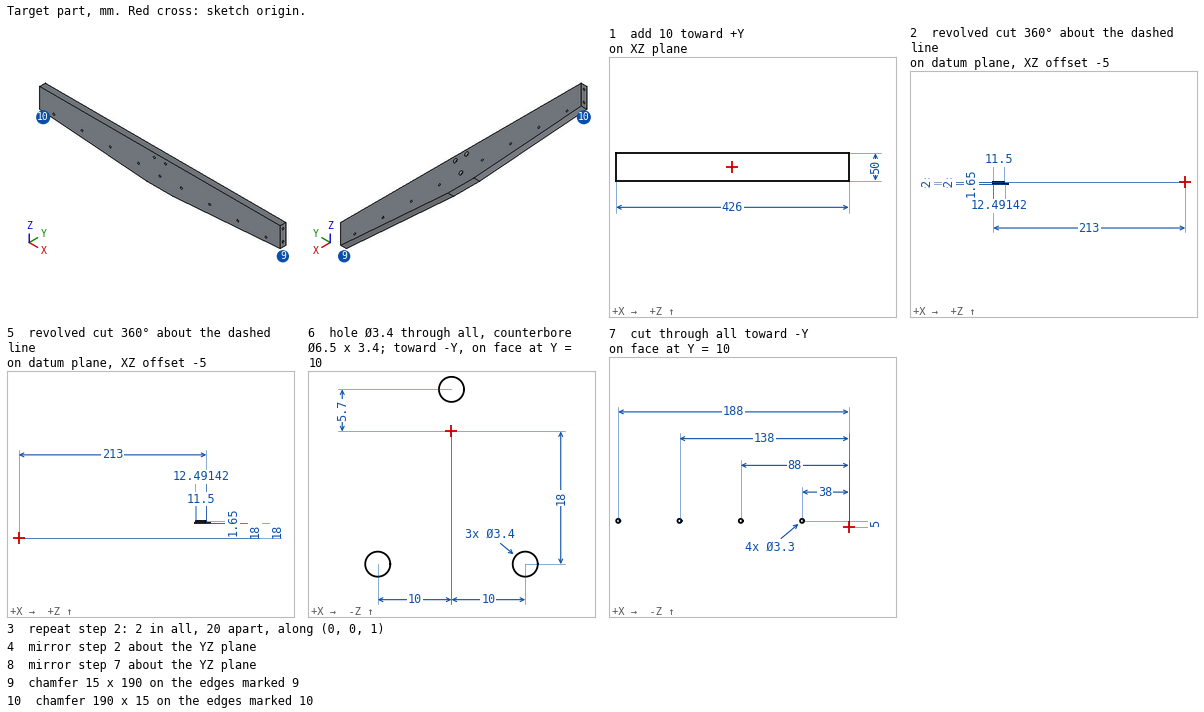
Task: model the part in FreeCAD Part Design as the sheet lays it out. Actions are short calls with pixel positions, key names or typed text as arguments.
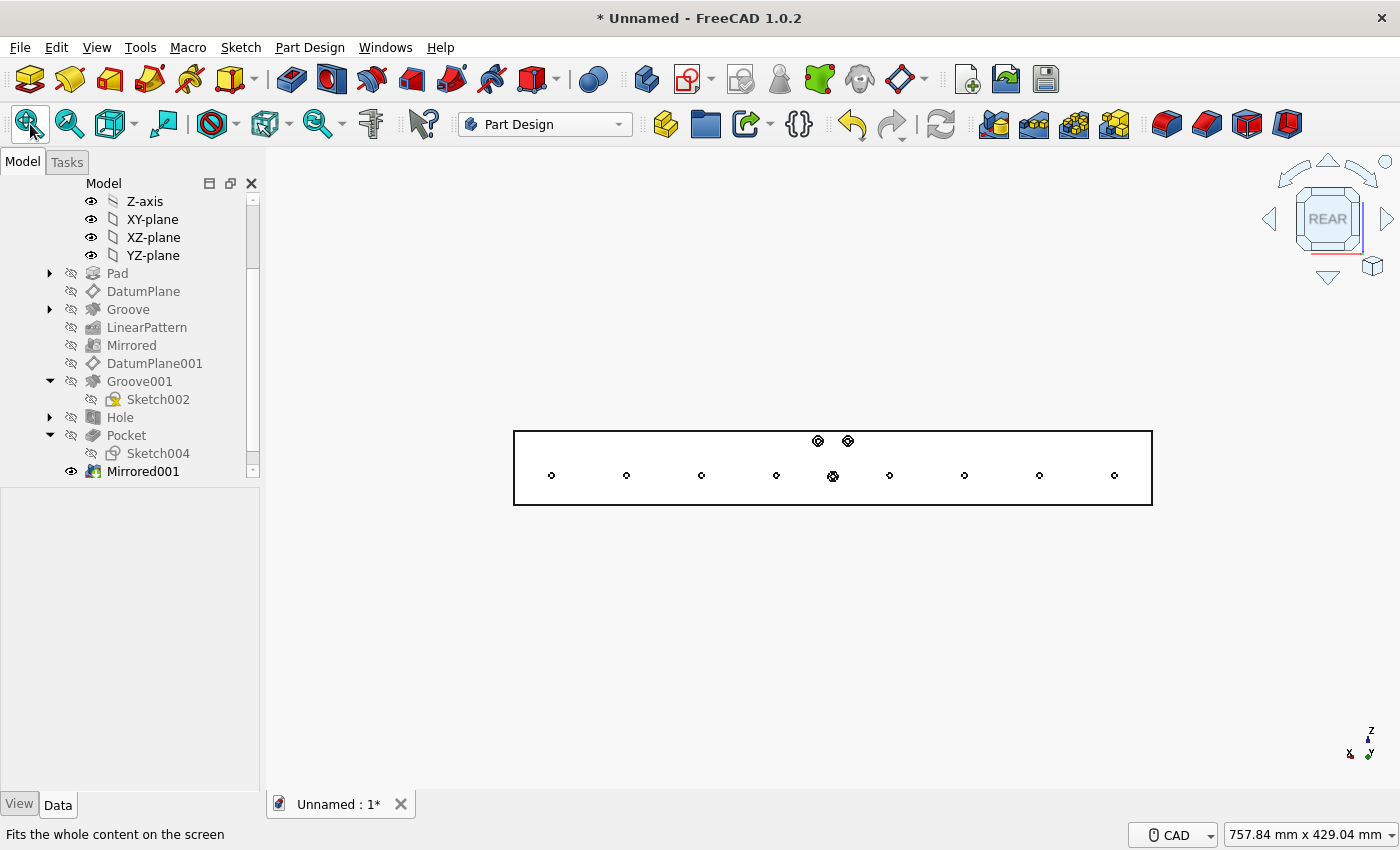
key(0)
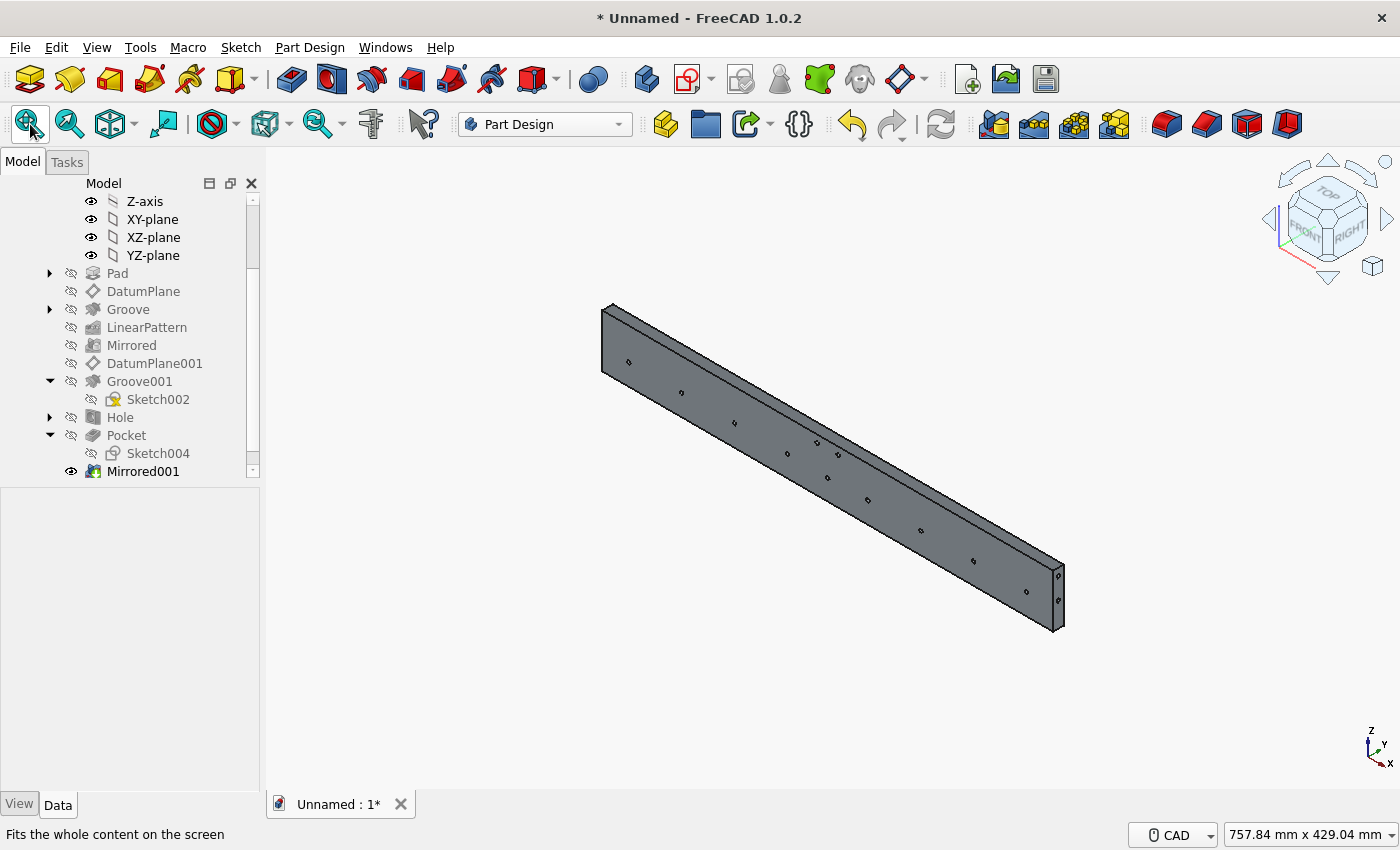
scroll(1058, 628, up, 5)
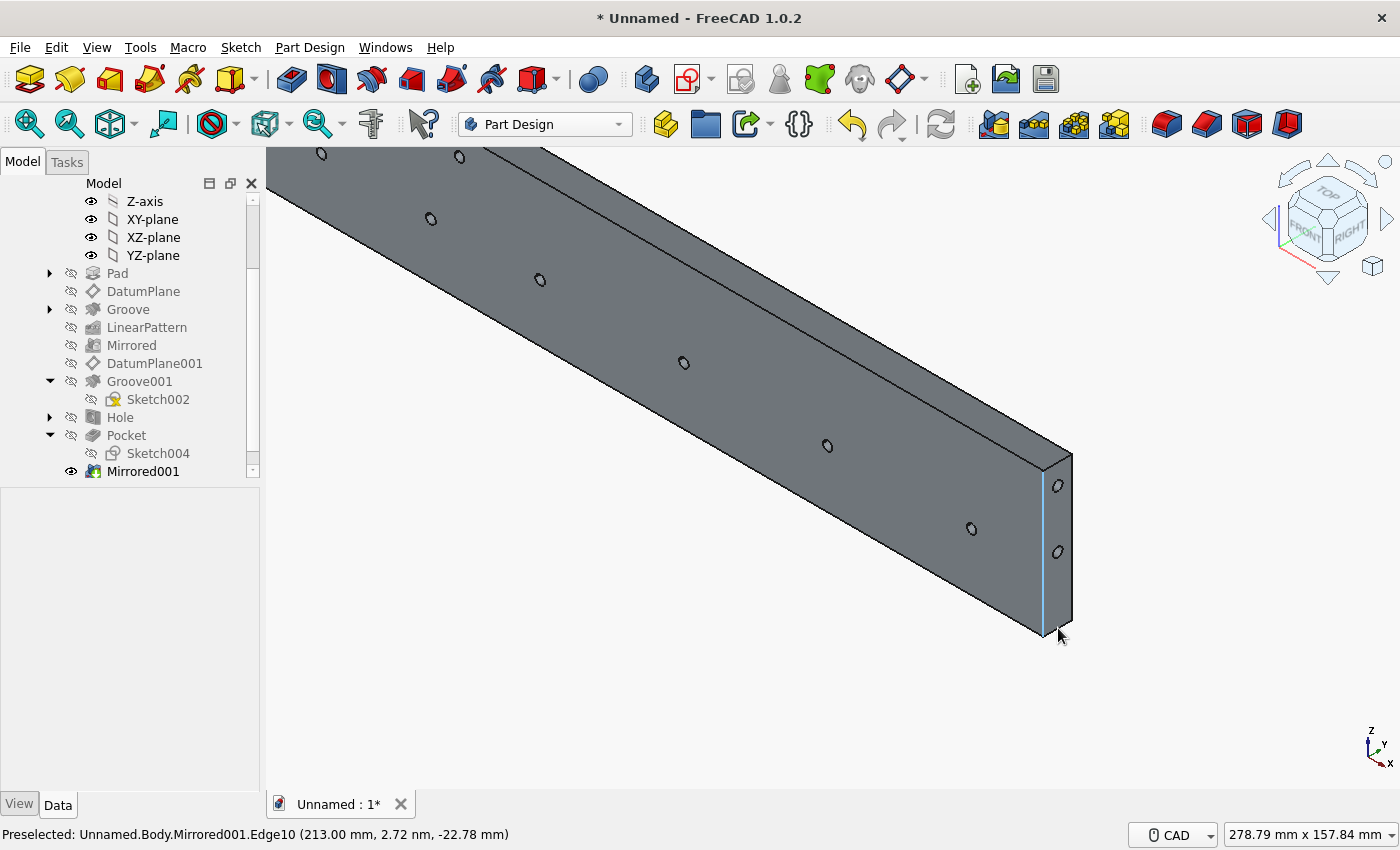
click(30, 124)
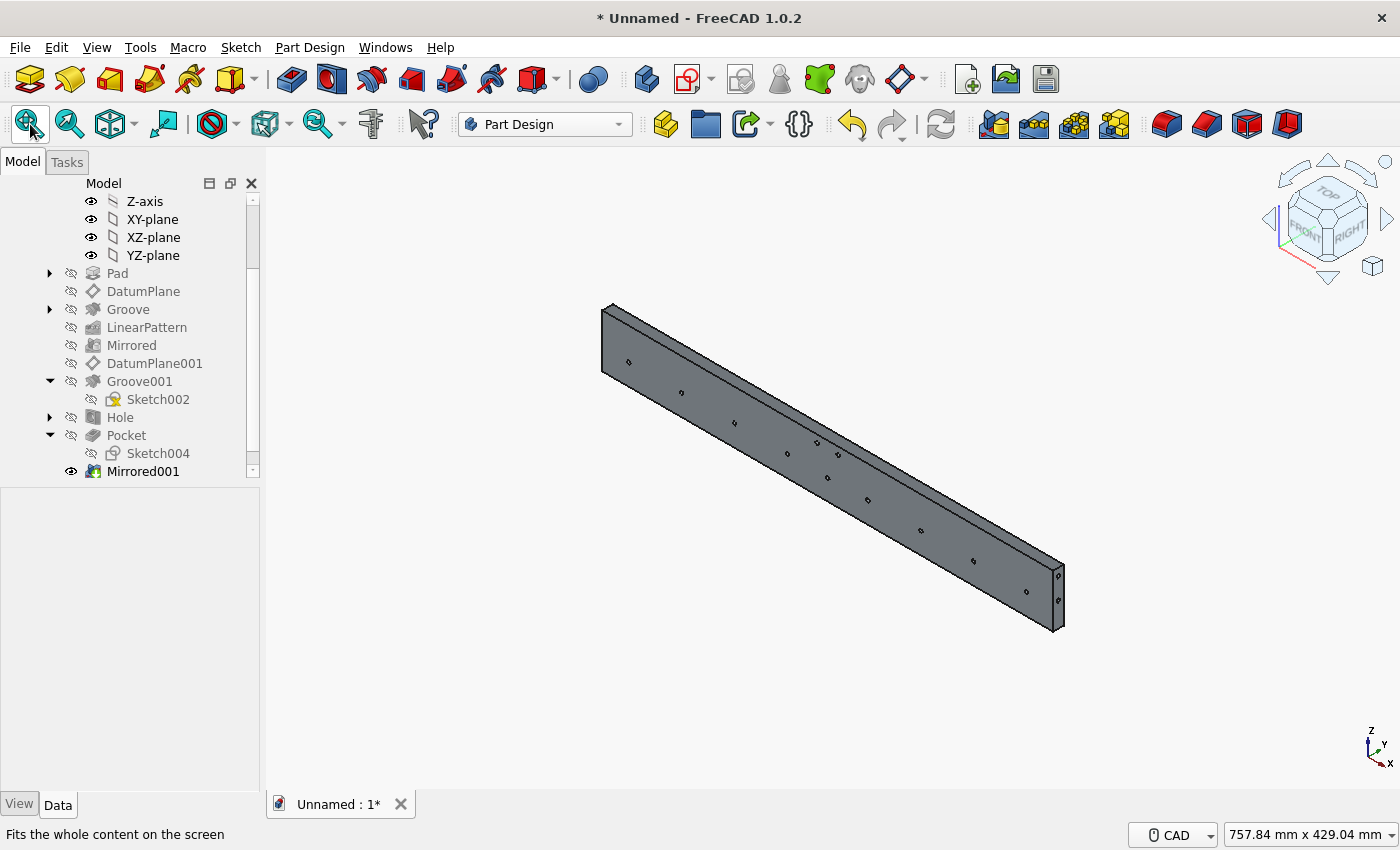
key(2)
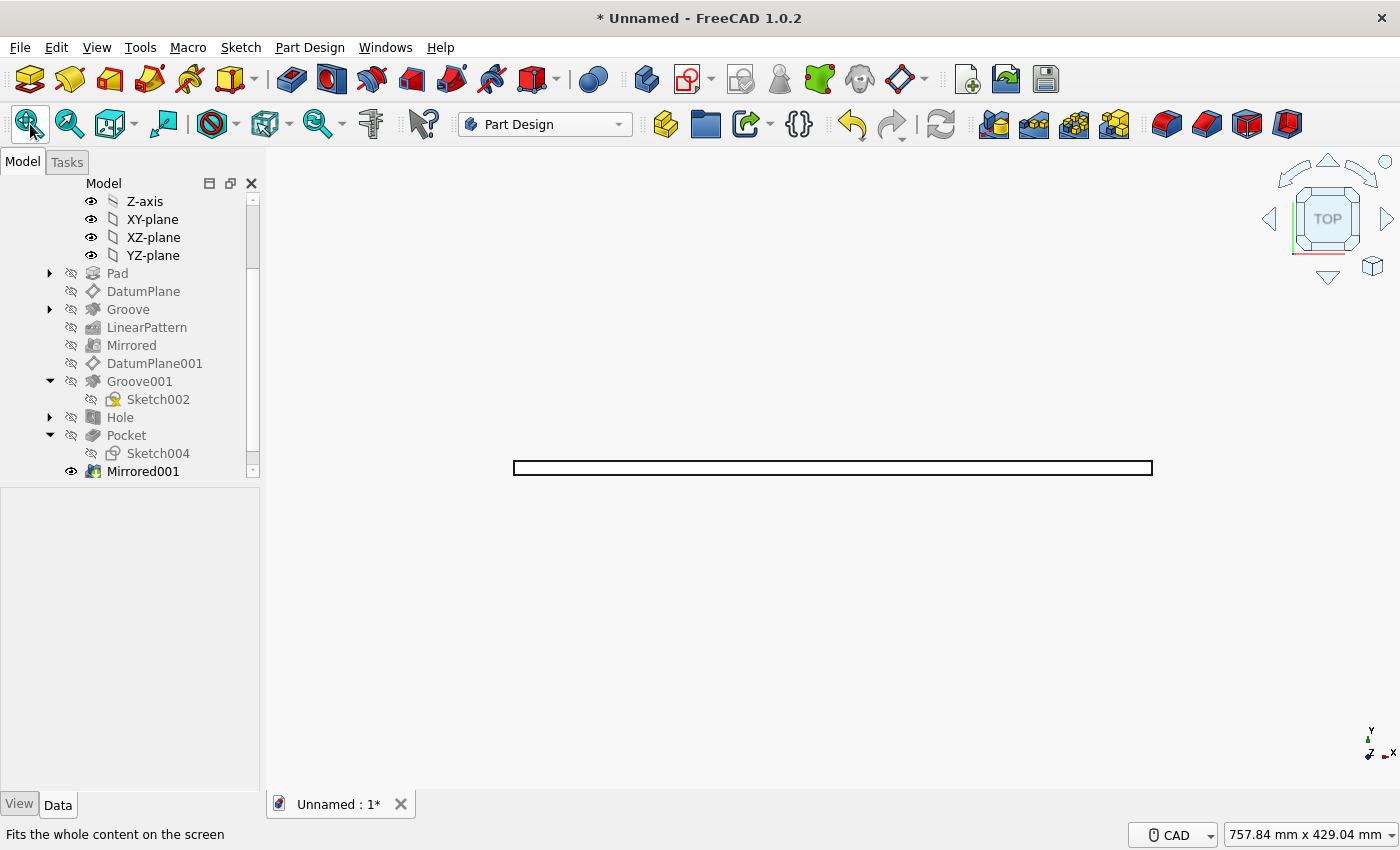
scroll(1152, 467, up, 5)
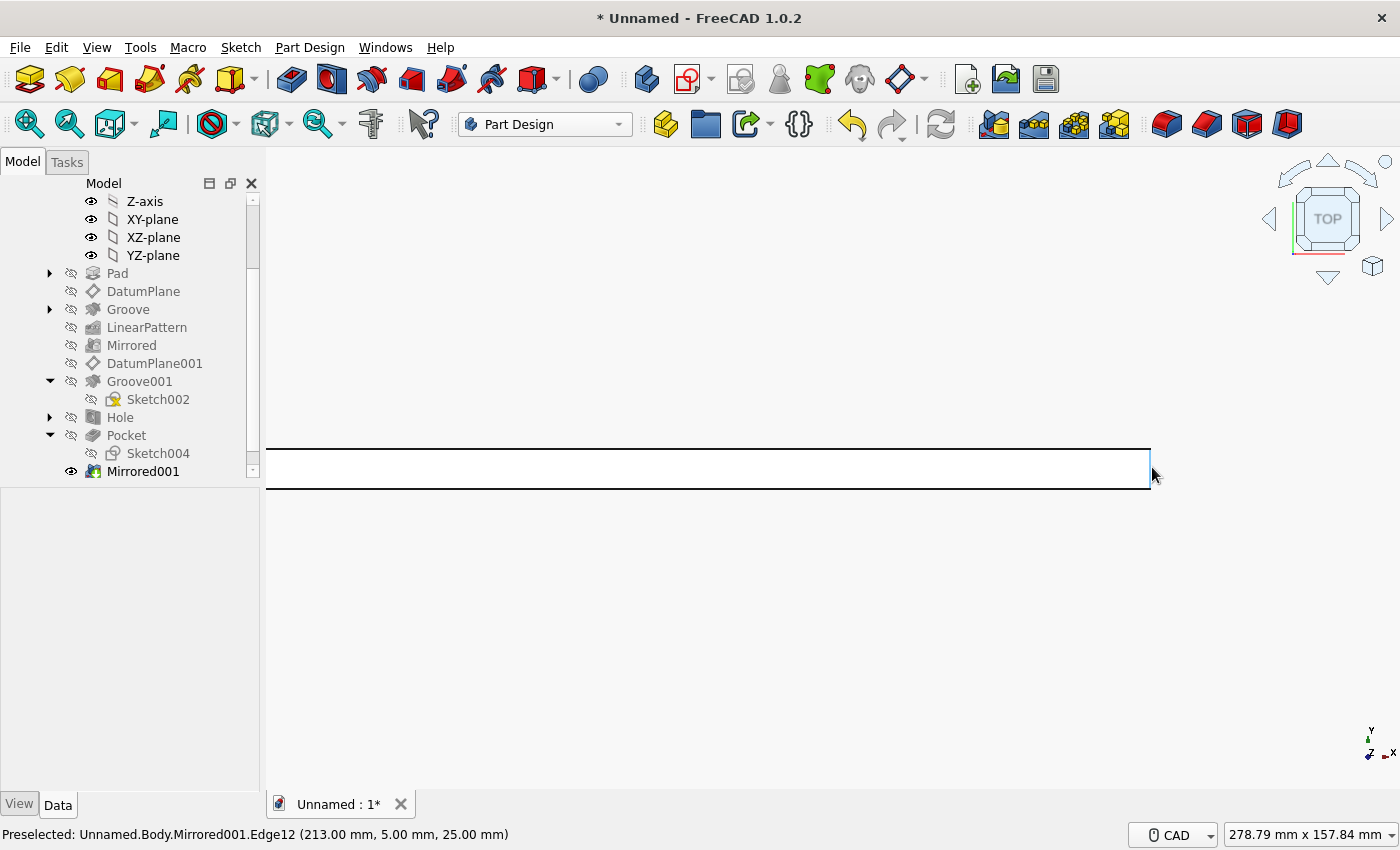
click(30, 124)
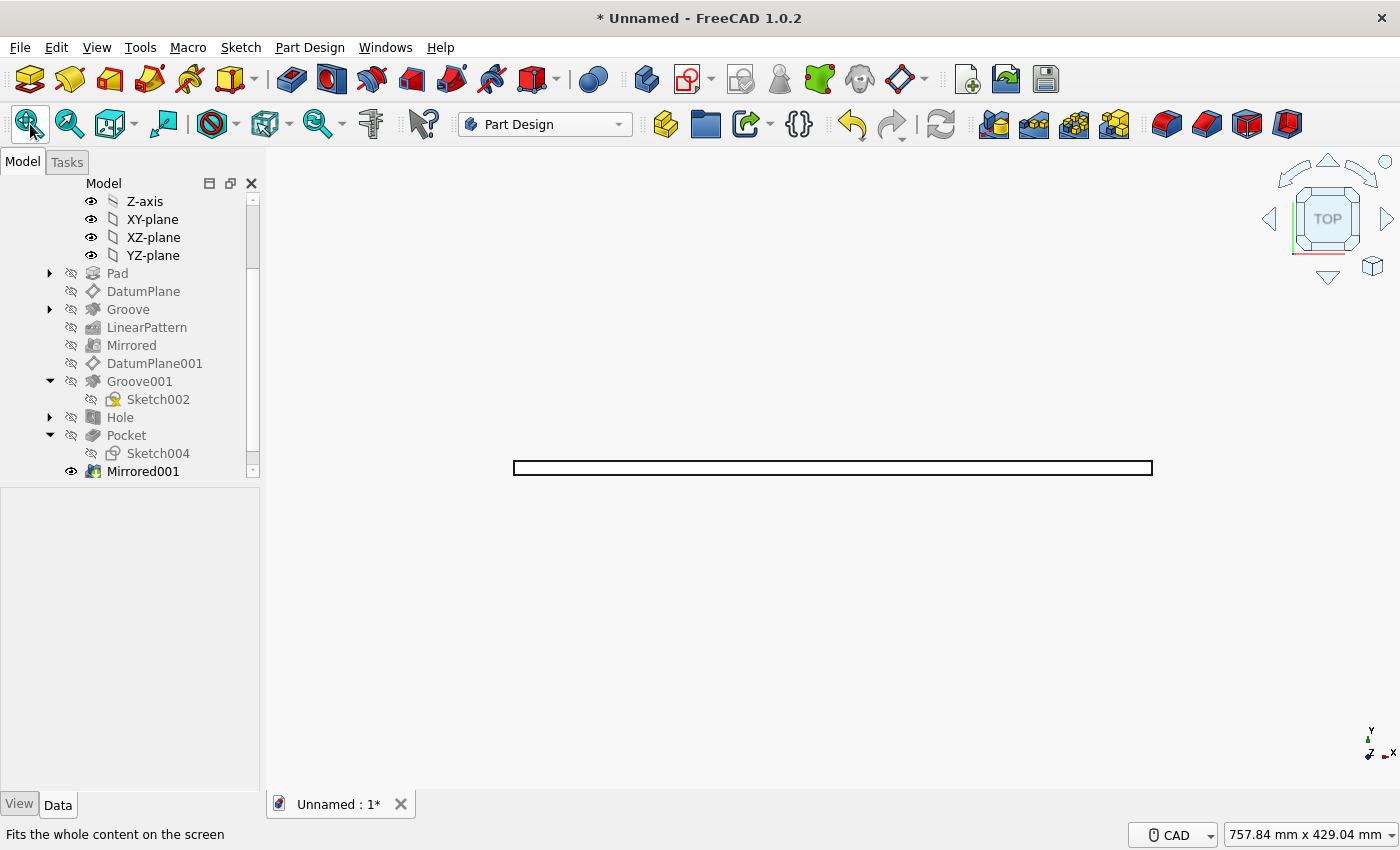
key(1)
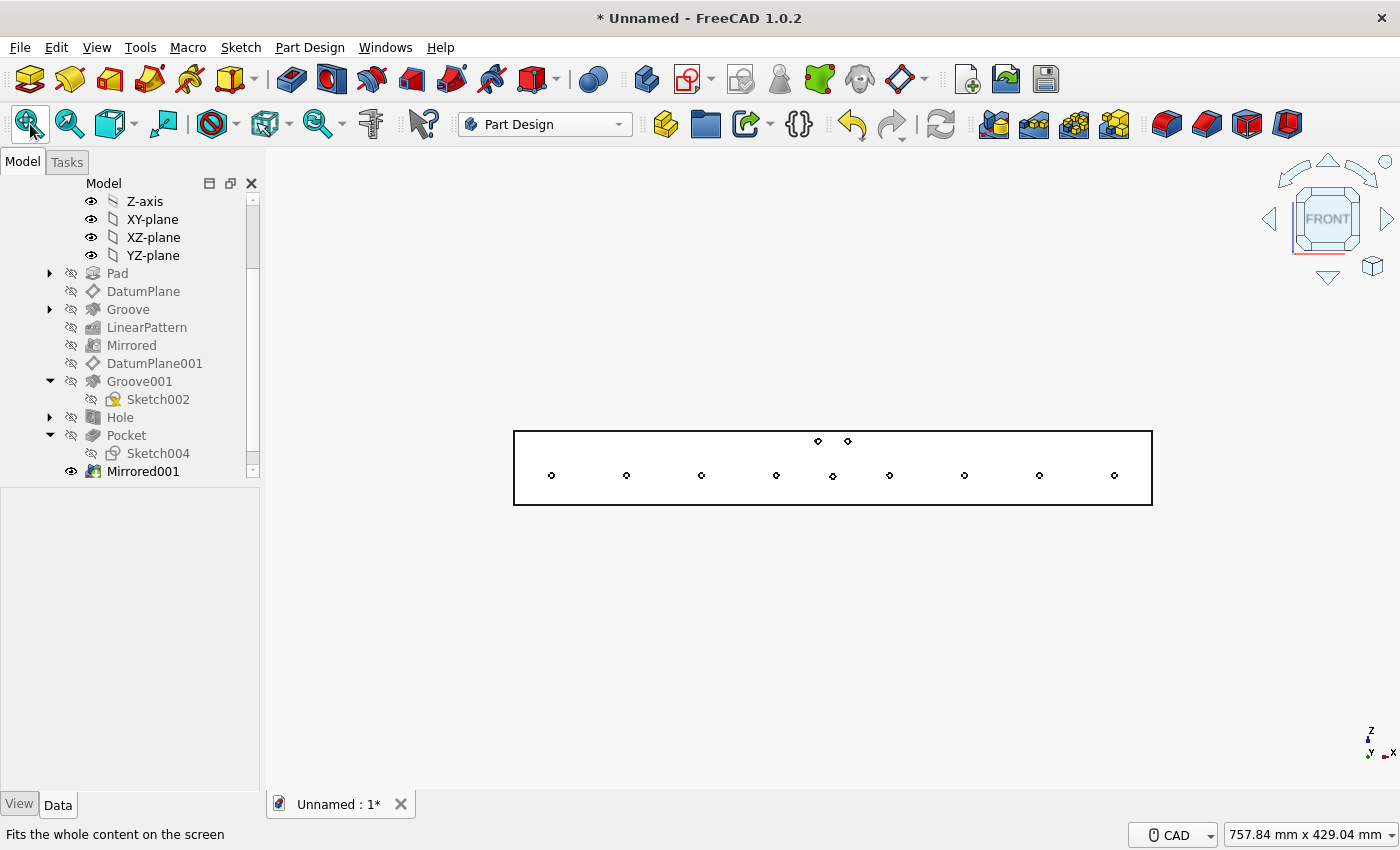
scroll(1152, 504, up, 5)